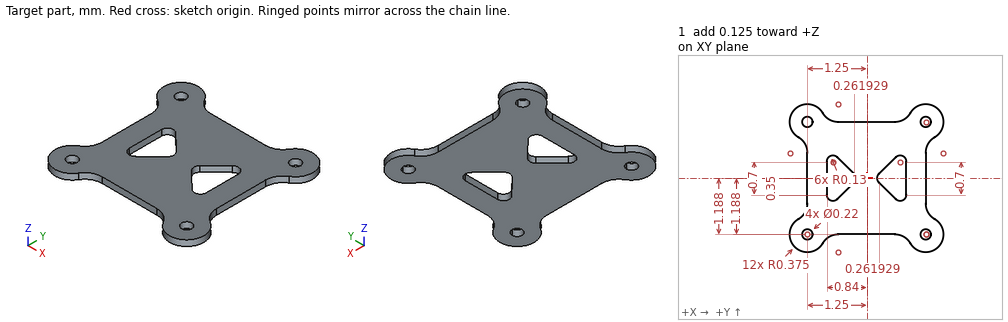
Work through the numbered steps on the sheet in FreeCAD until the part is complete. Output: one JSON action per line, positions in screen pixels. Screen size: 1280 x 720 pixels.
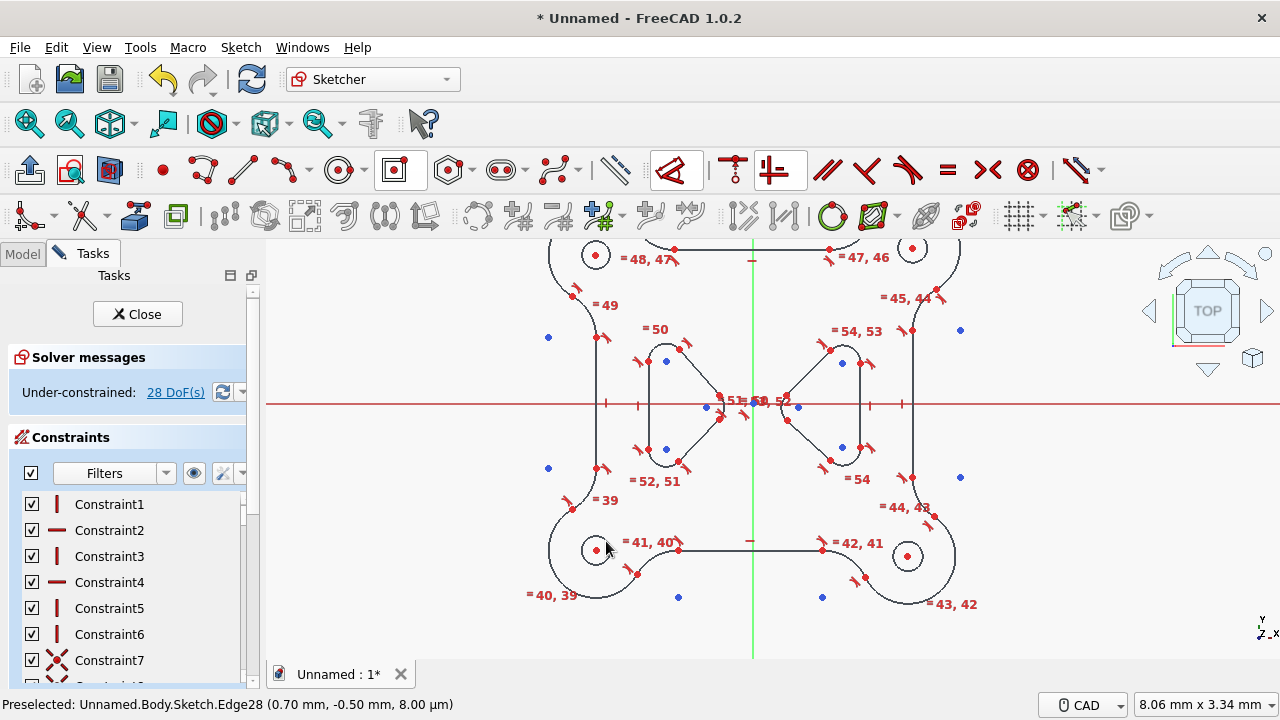
{"action": "left_click", "coordinate": [606, 540]}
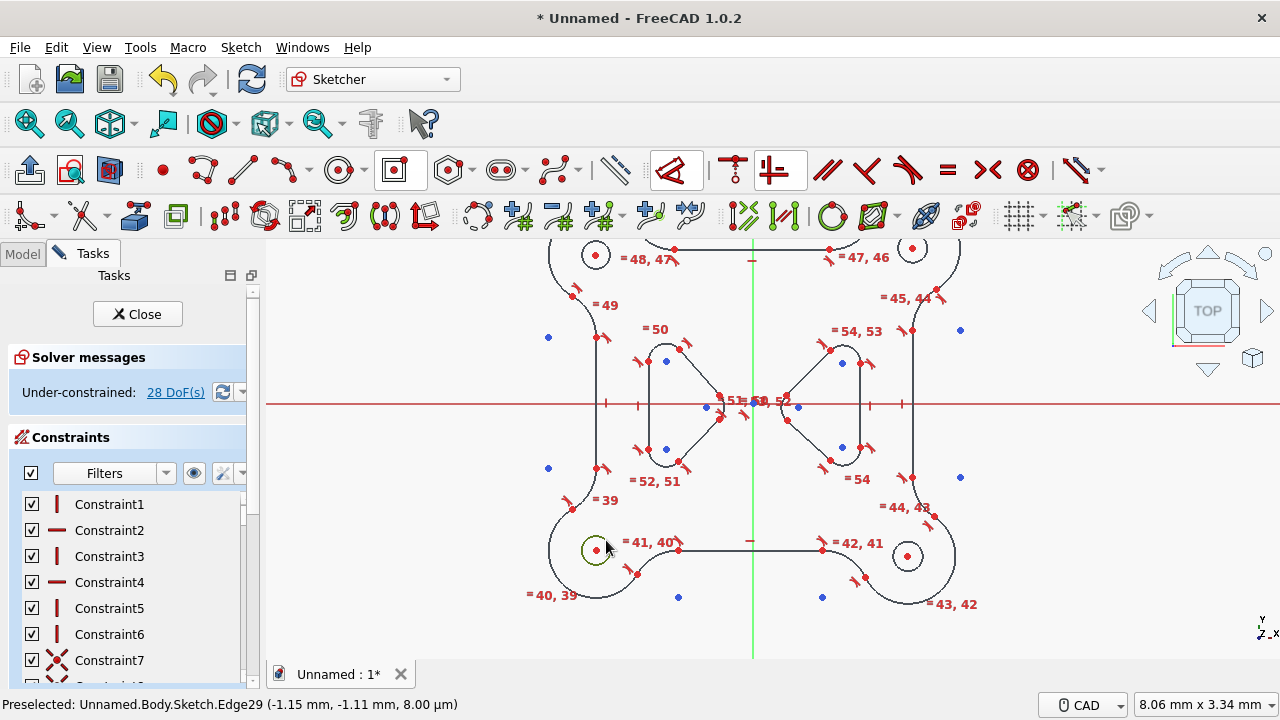
{"action": "left_click", "coordinate": [918, 546]}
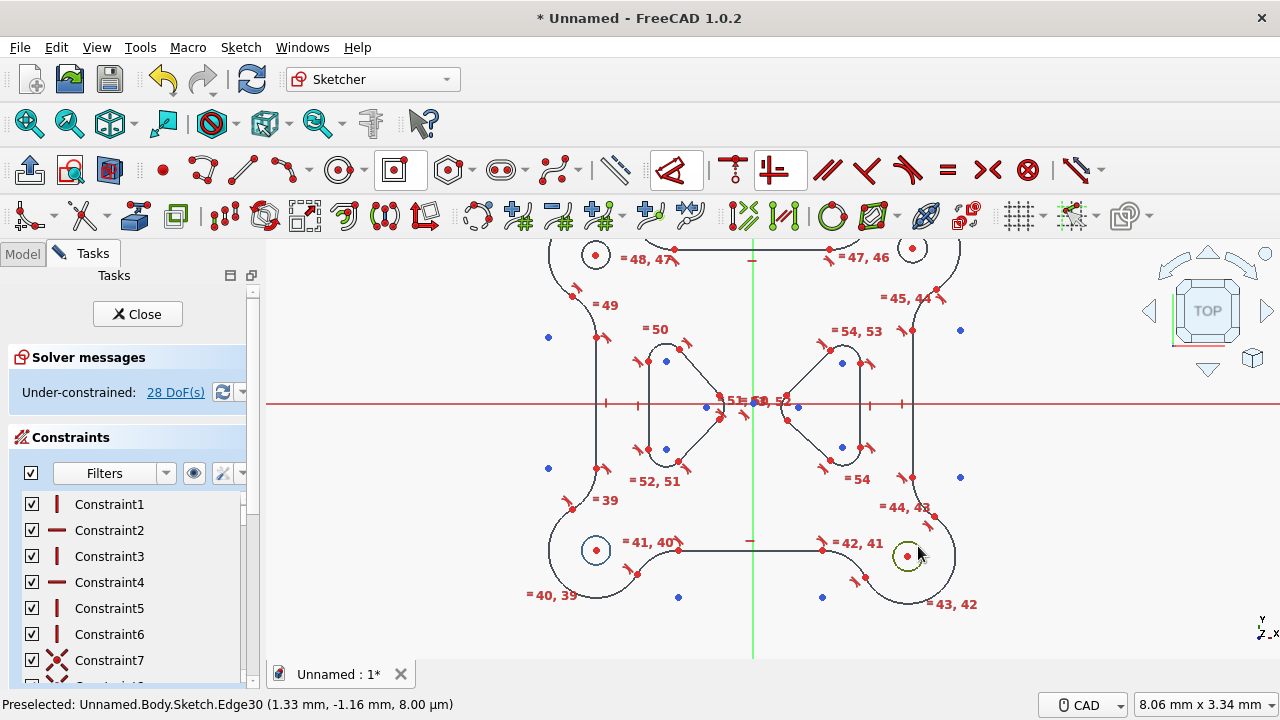
{"action": "left_click", "coordinate": [596, 269]}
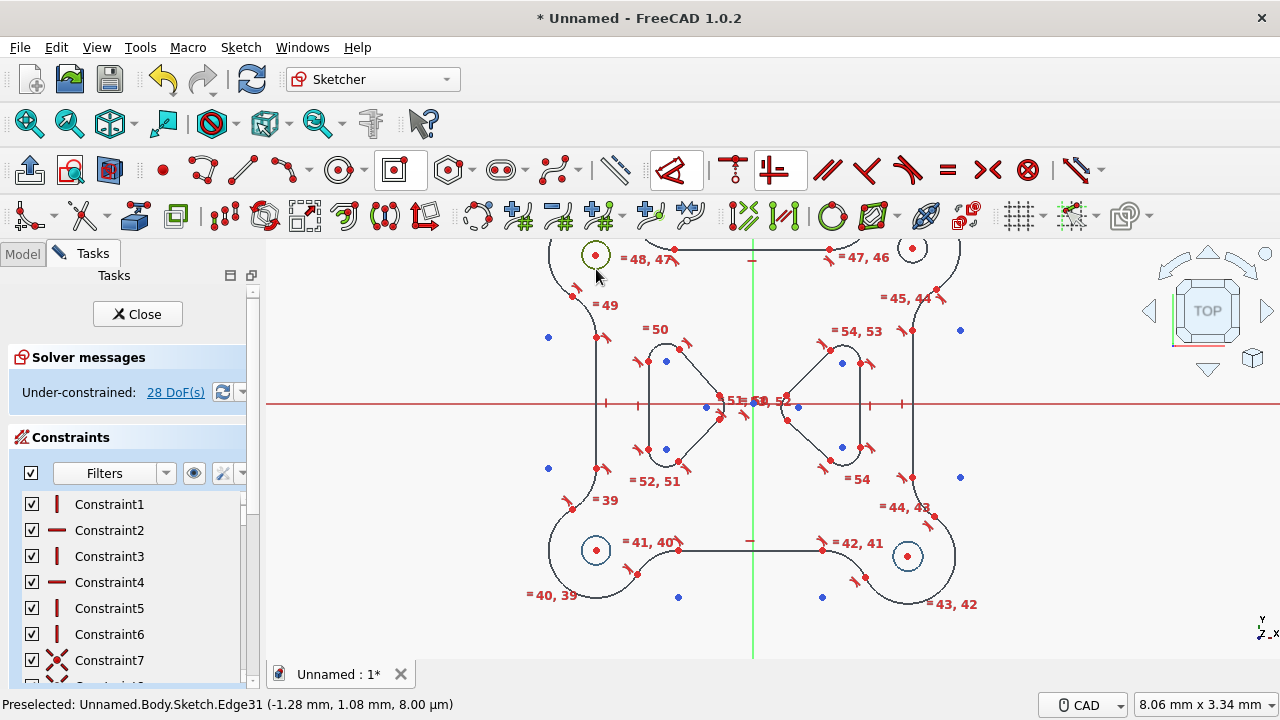
{"action": "scroll", "coordinate": [605, 541], "scroll_direction": "down", "scroll_amount": 2}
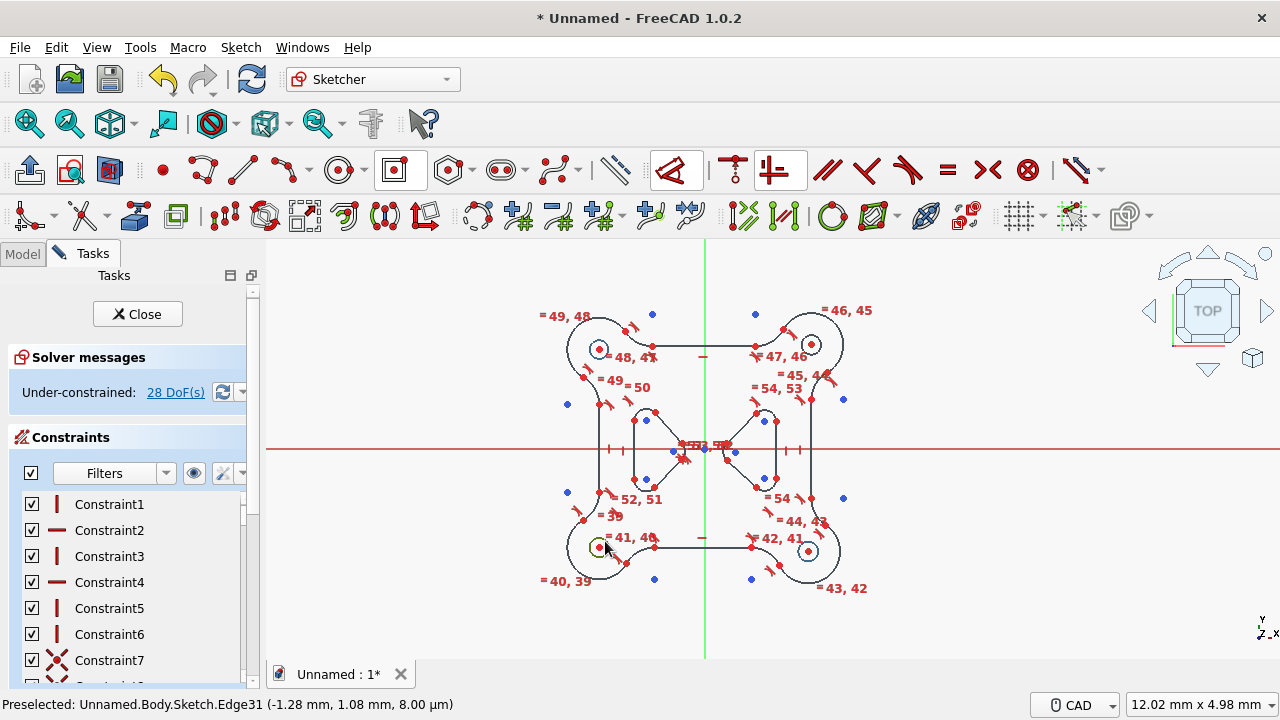
{"action": "scroll", "coordinate": [818, 338], "scroll_direction": "up", "scroll_amount": 2}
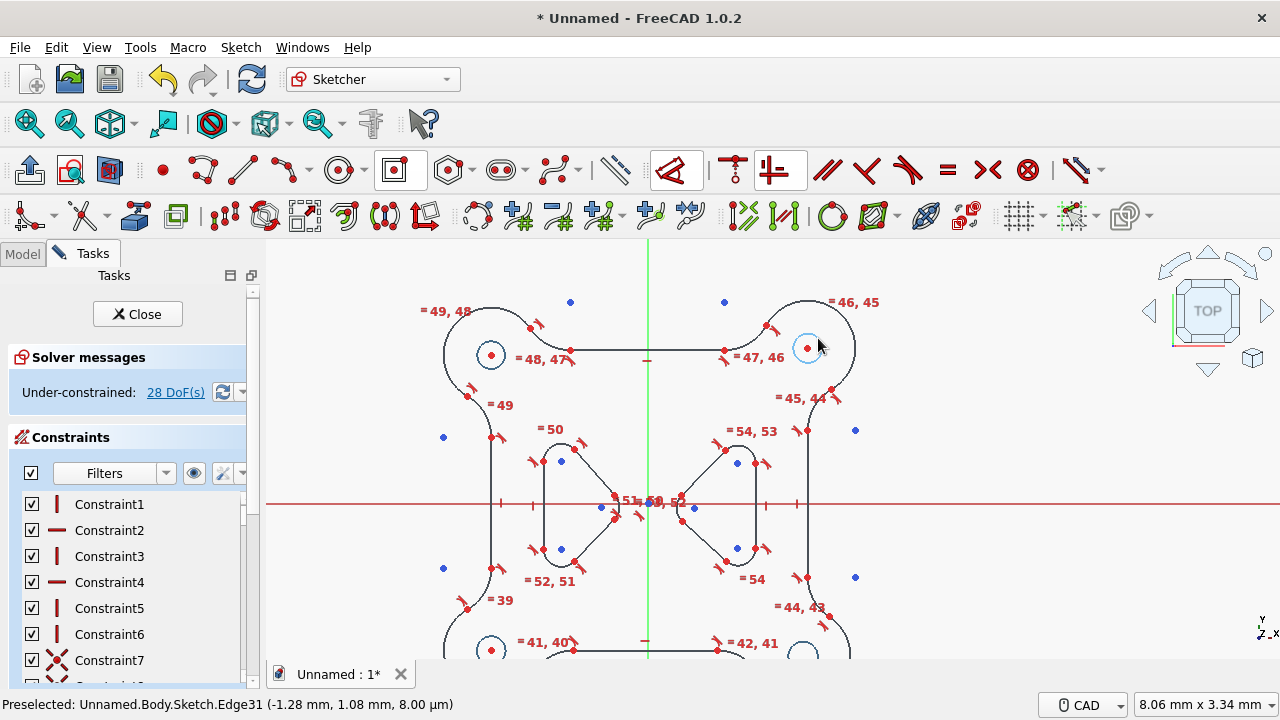
{"action": "left_click", "coordinate": [818, 338]}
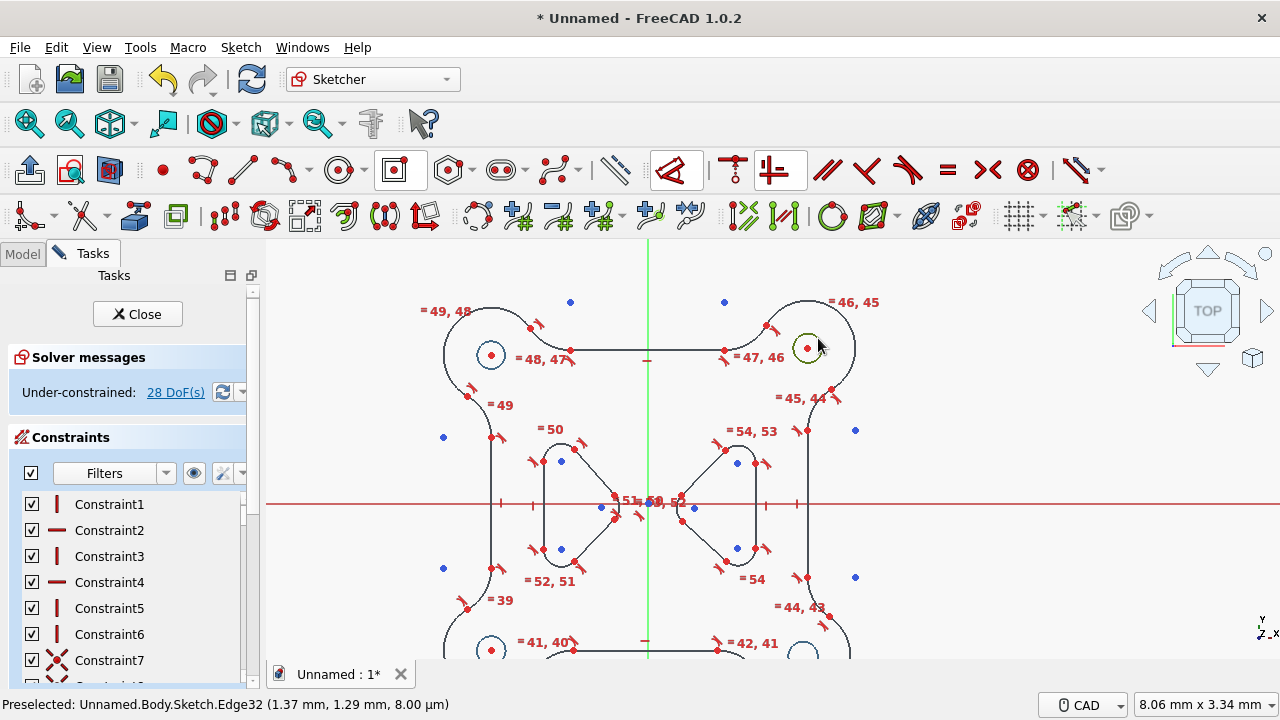
{"action": "left_click", "coordinate": [948, 170]}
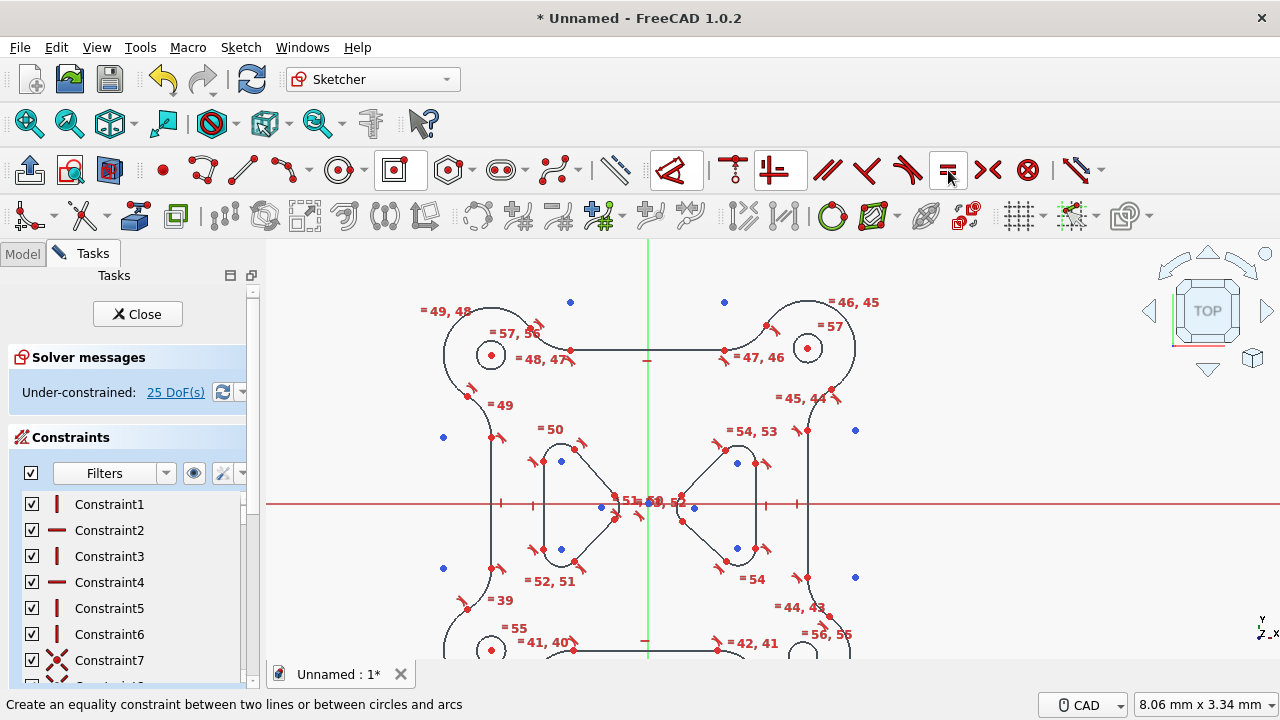
{"action": "left_click", "coordinate": [602, 507]}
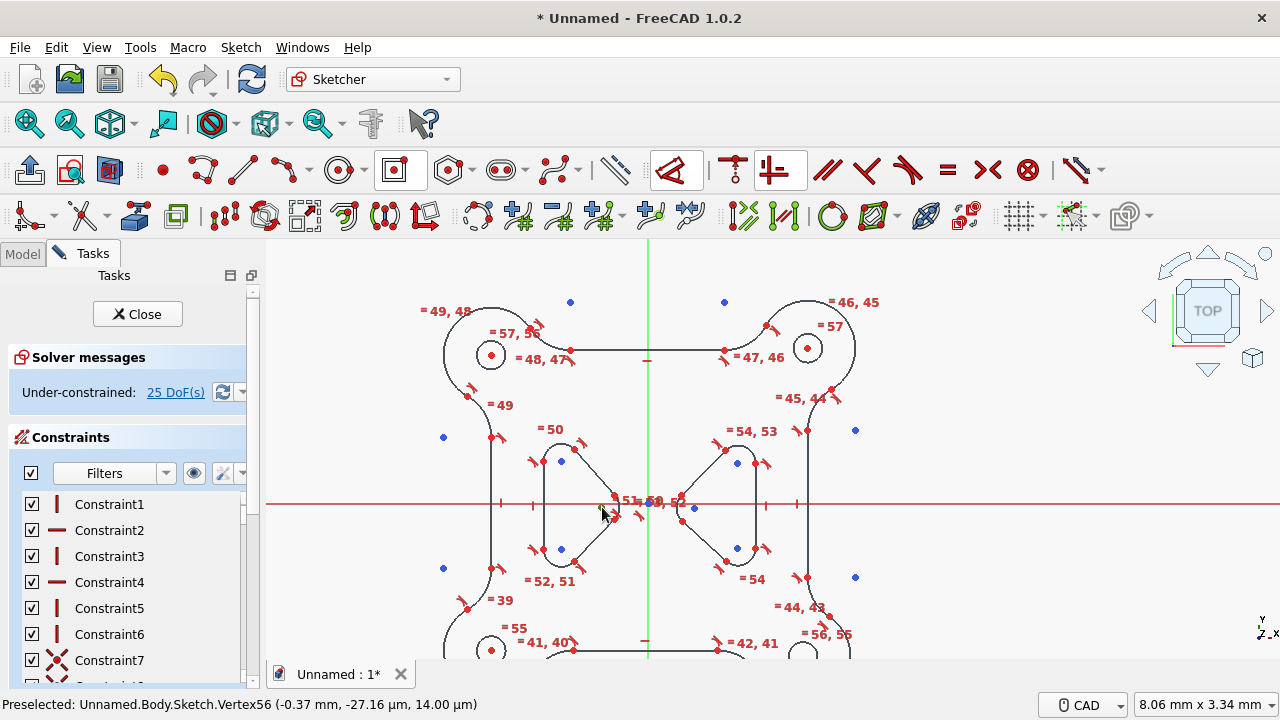
{"action": "left_click", "coordinate": [353, 504]}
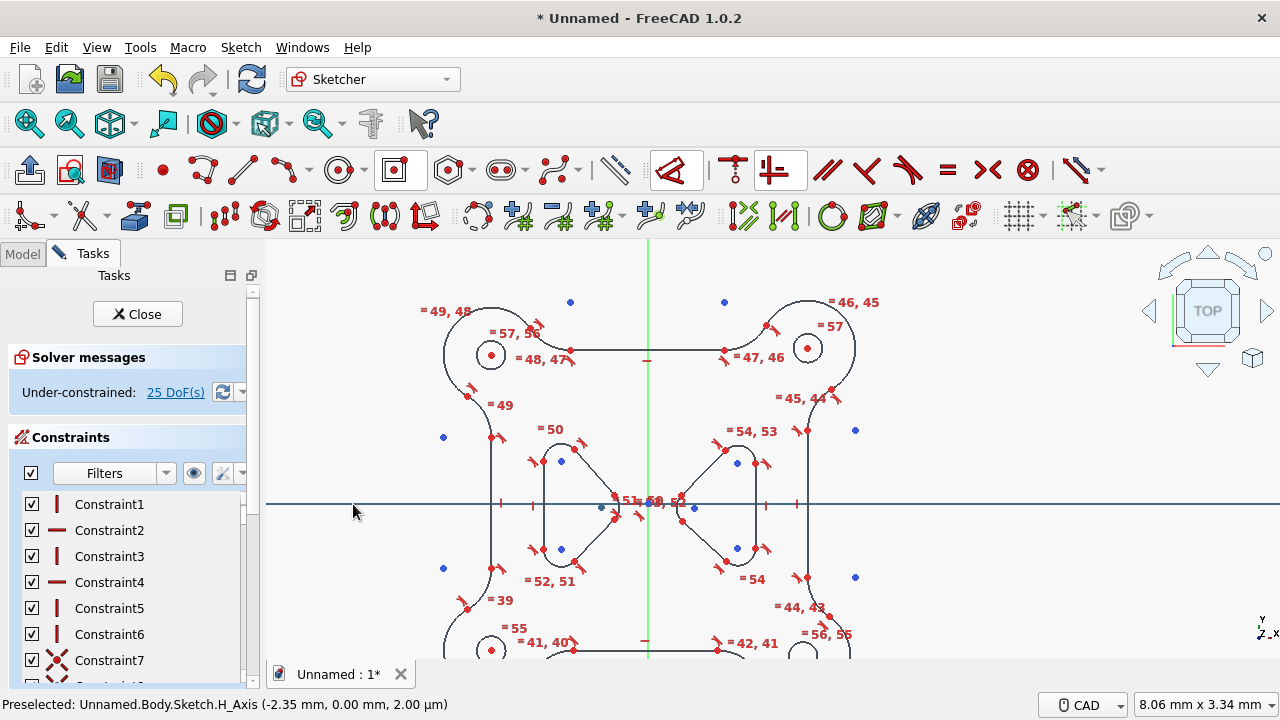
{"action": "left_click", "coordinate": [734, 170]}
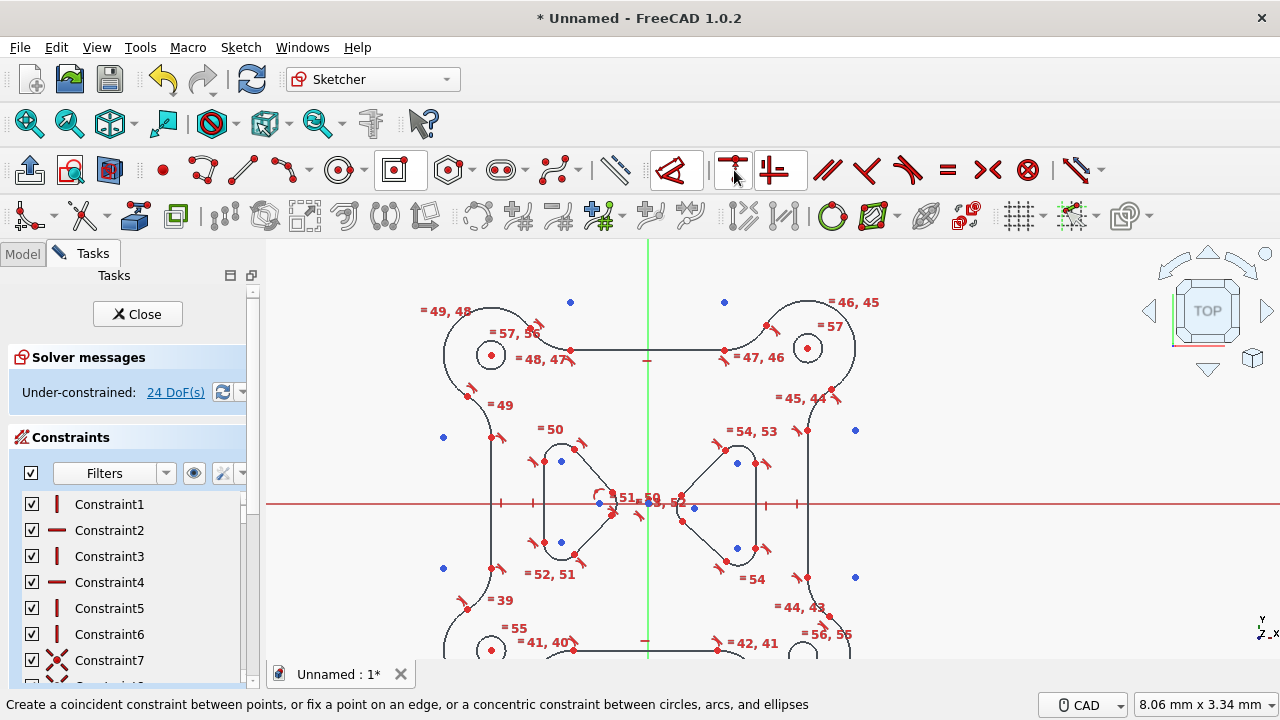
{"action": "left_click", "coordinate": [694, 508]}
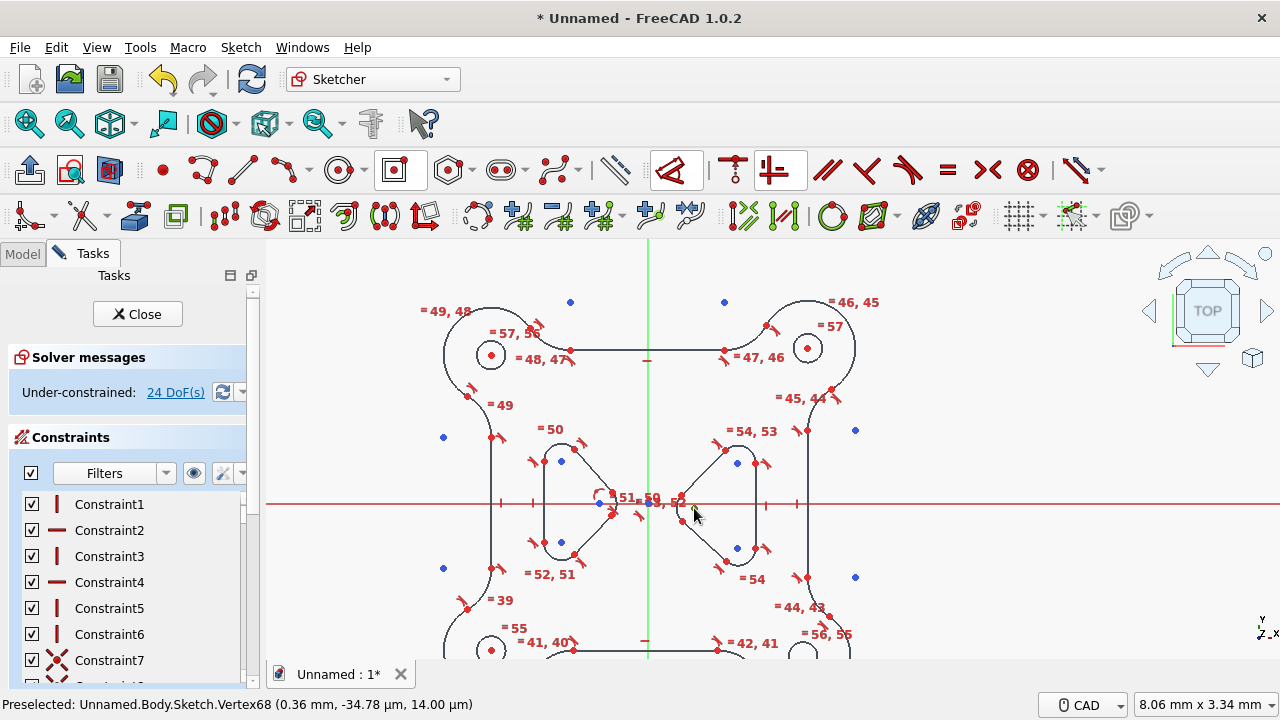
{"action": "left_click", "coordinate": [353, 504]}